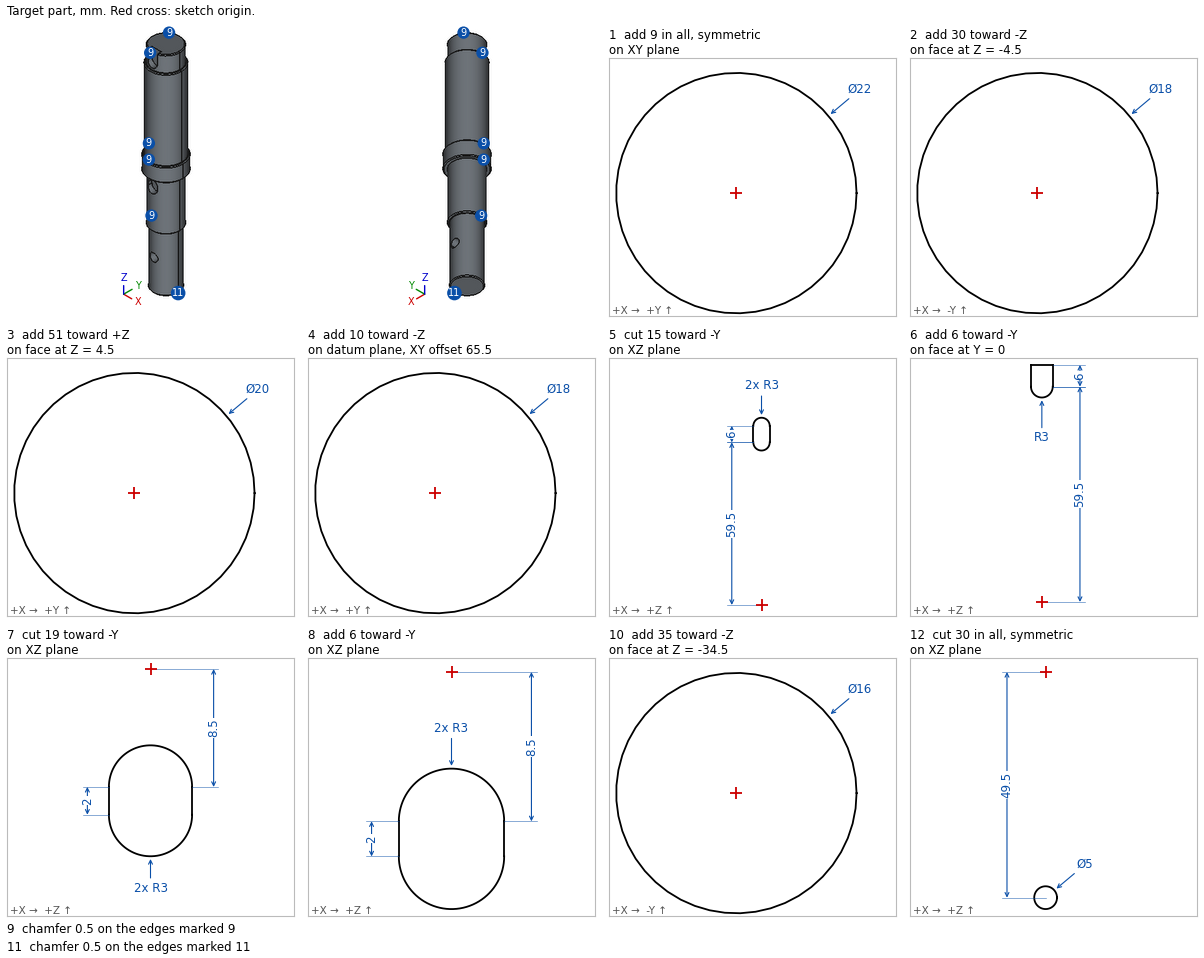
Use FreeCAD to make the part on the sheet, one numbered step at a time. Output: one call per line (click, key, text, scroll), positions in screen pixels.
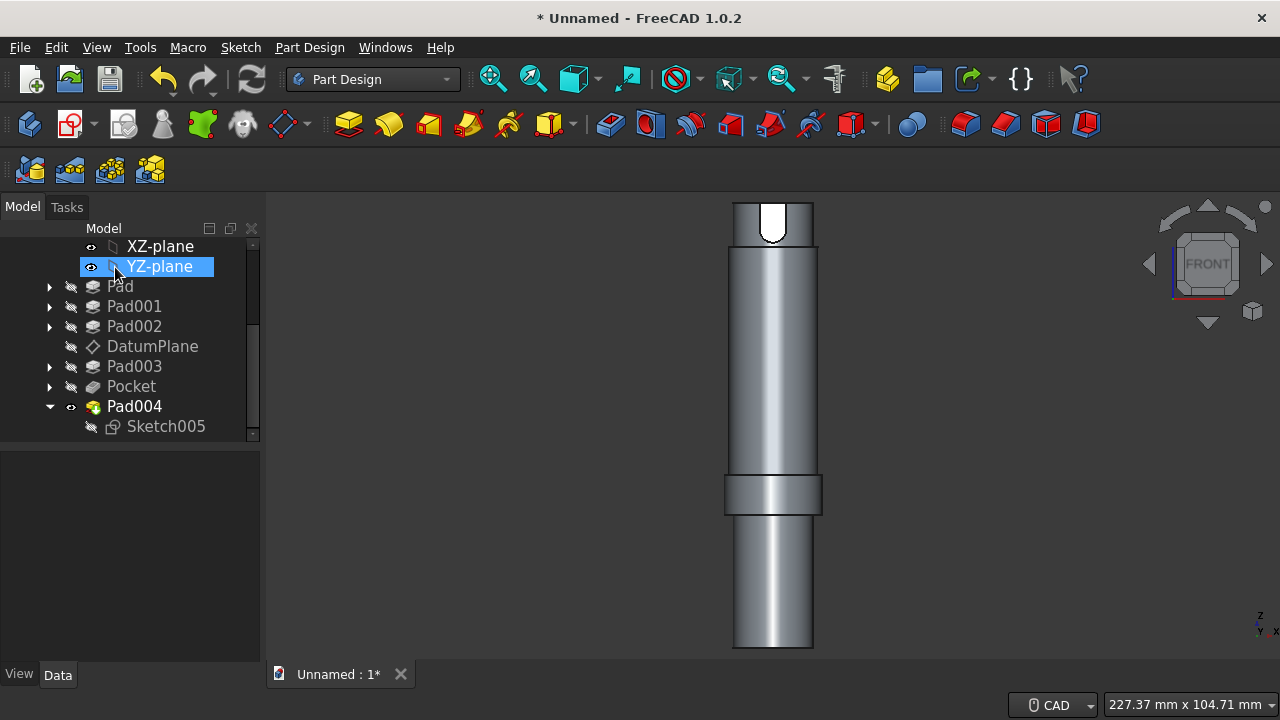
click(70, 124)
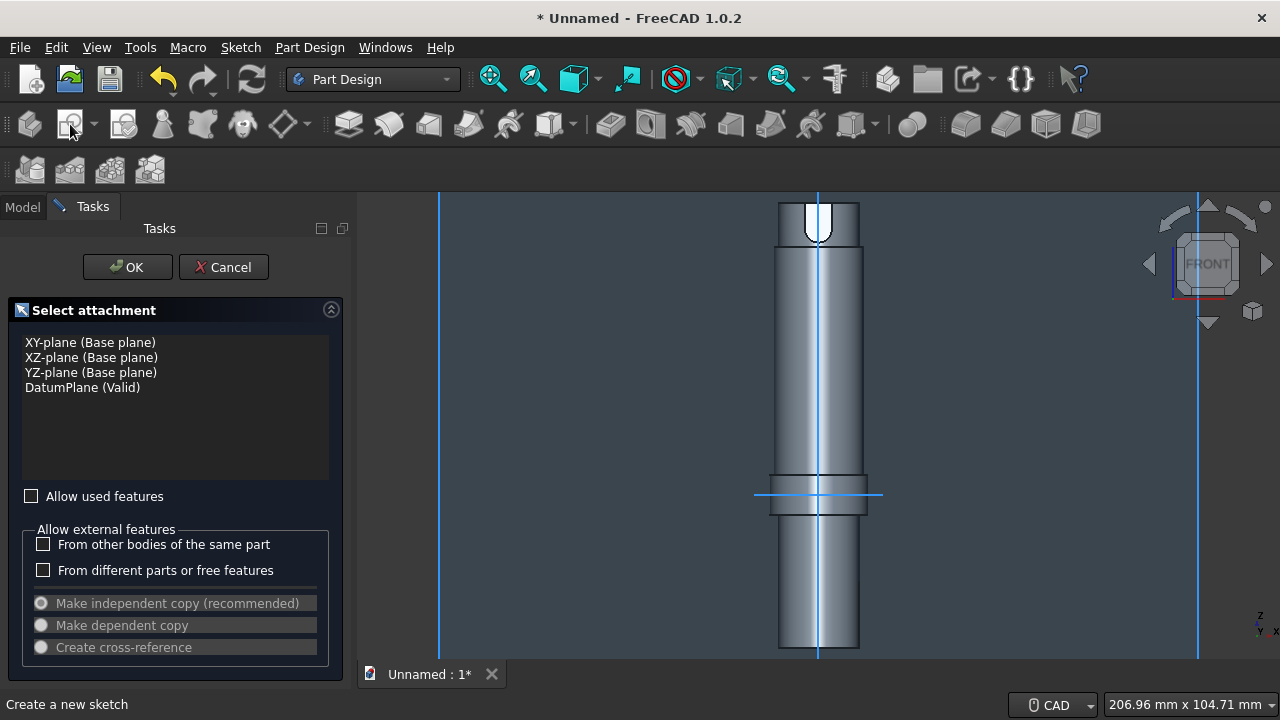
click(82, 358)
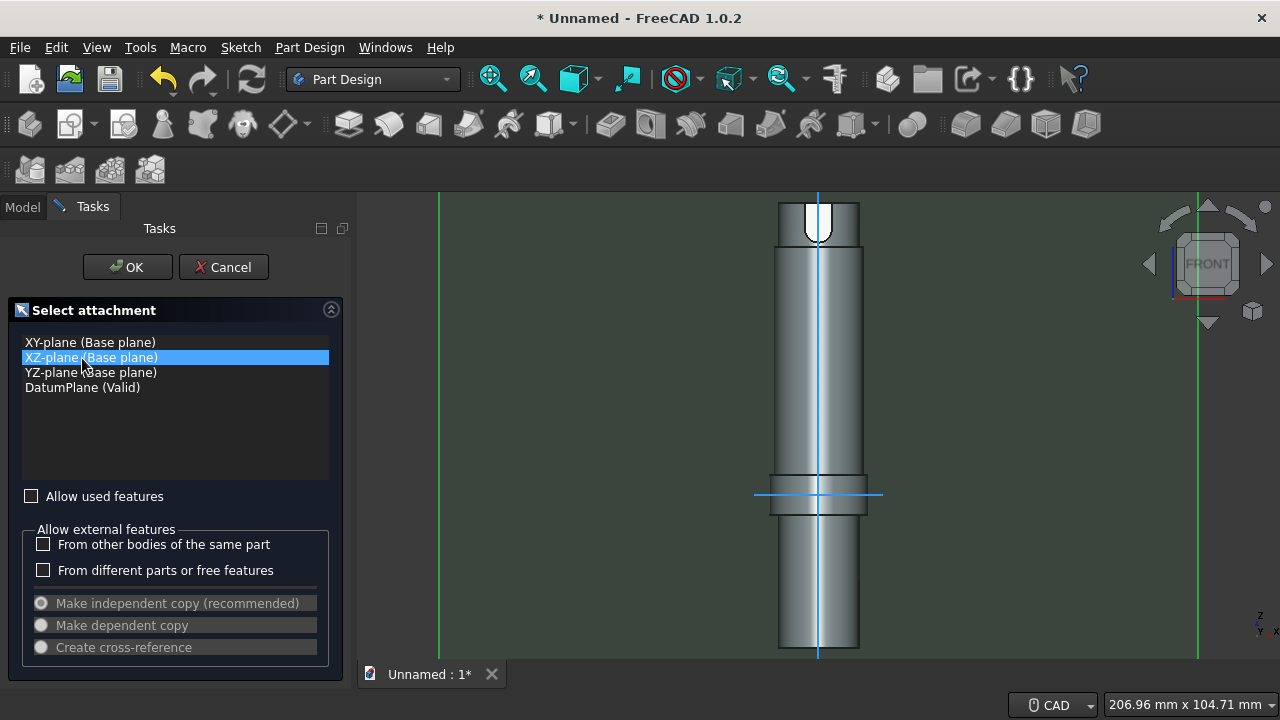
click(128, 267)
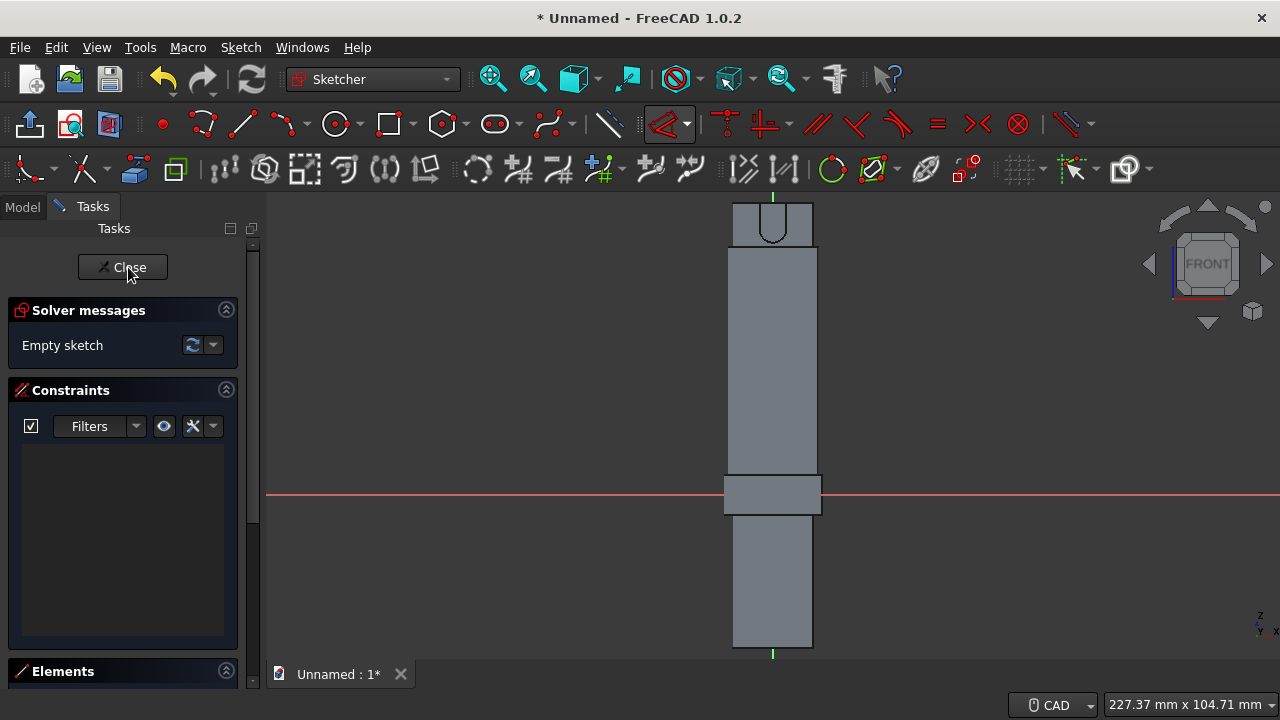
click(110, 124)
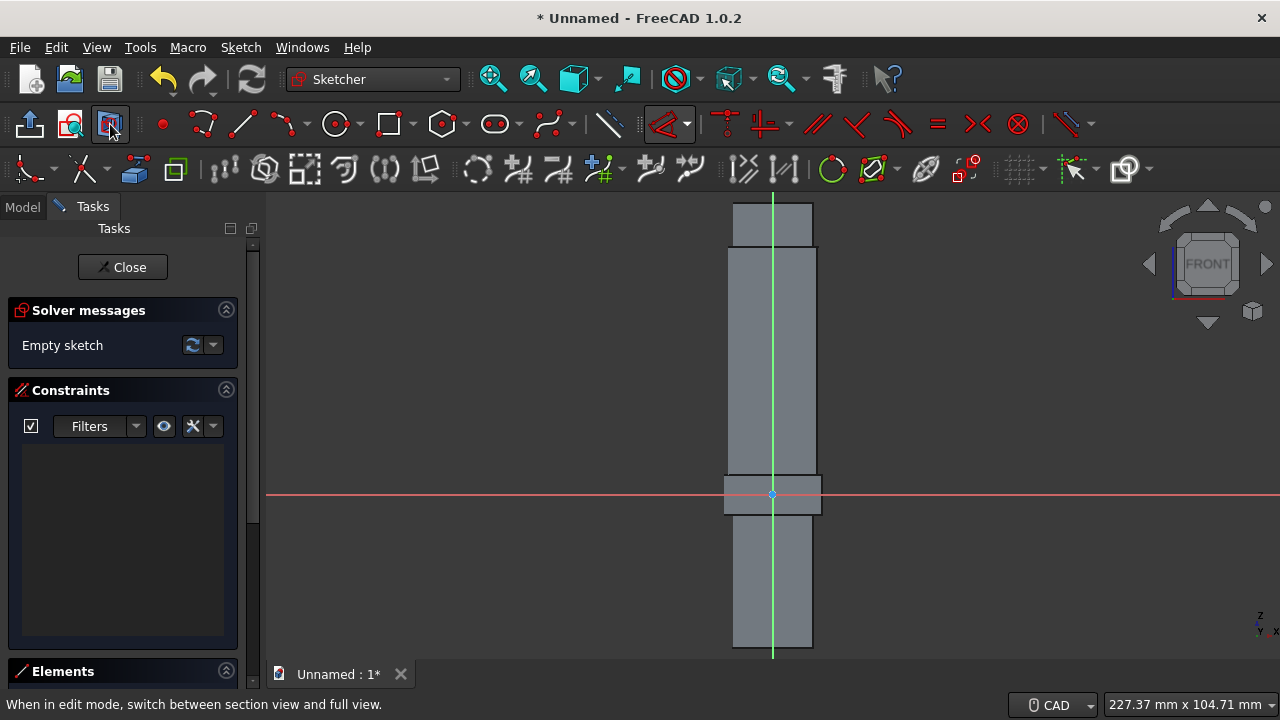
scroll(790, 550, up, 8)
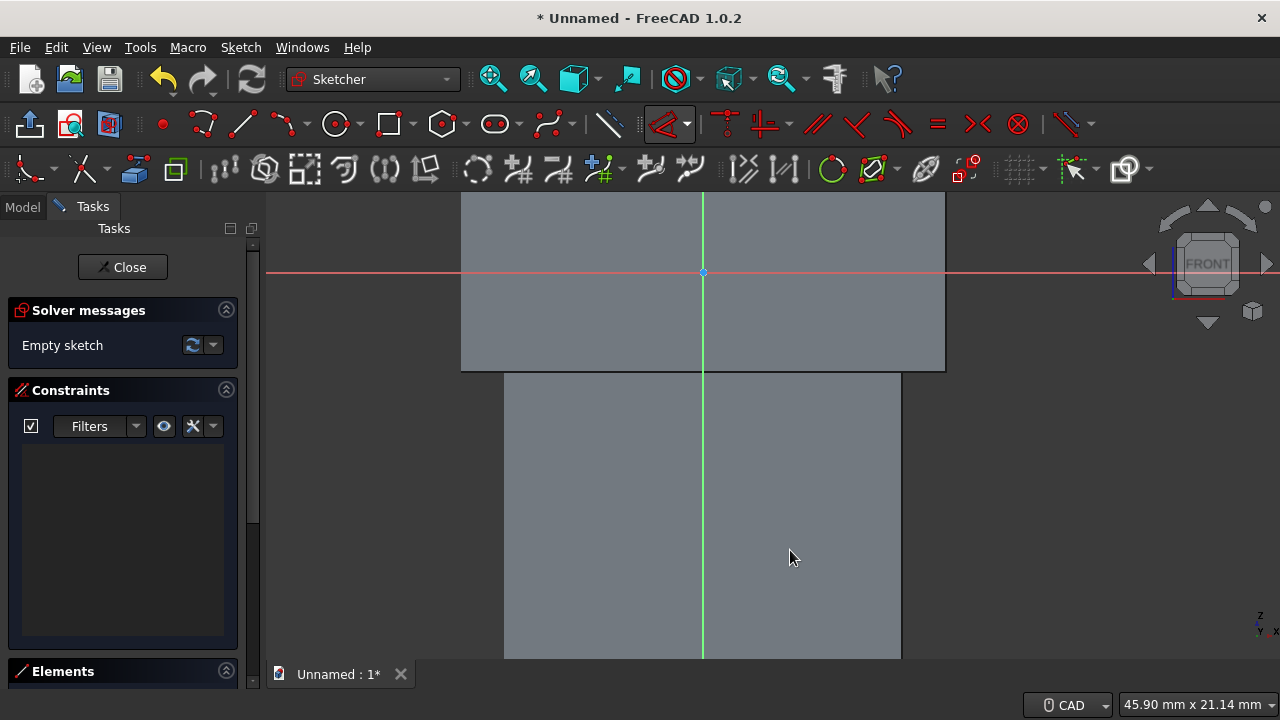
click(496, 124)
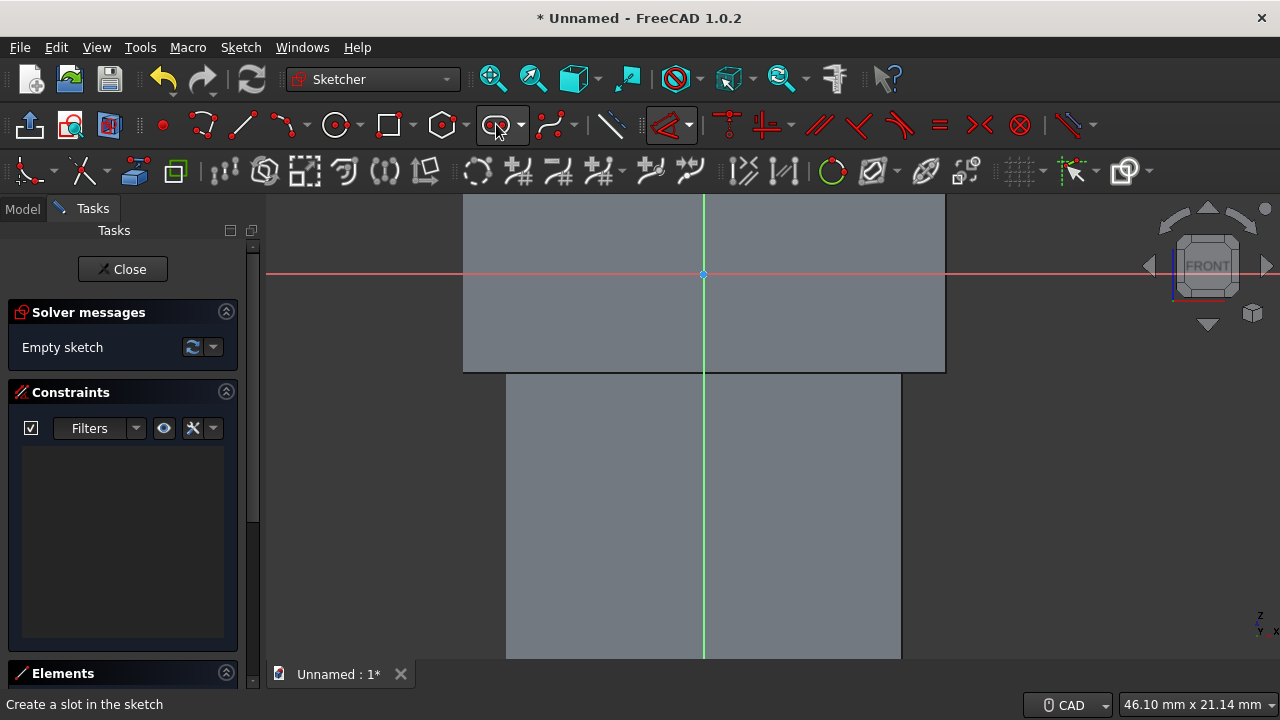
click(704, 505)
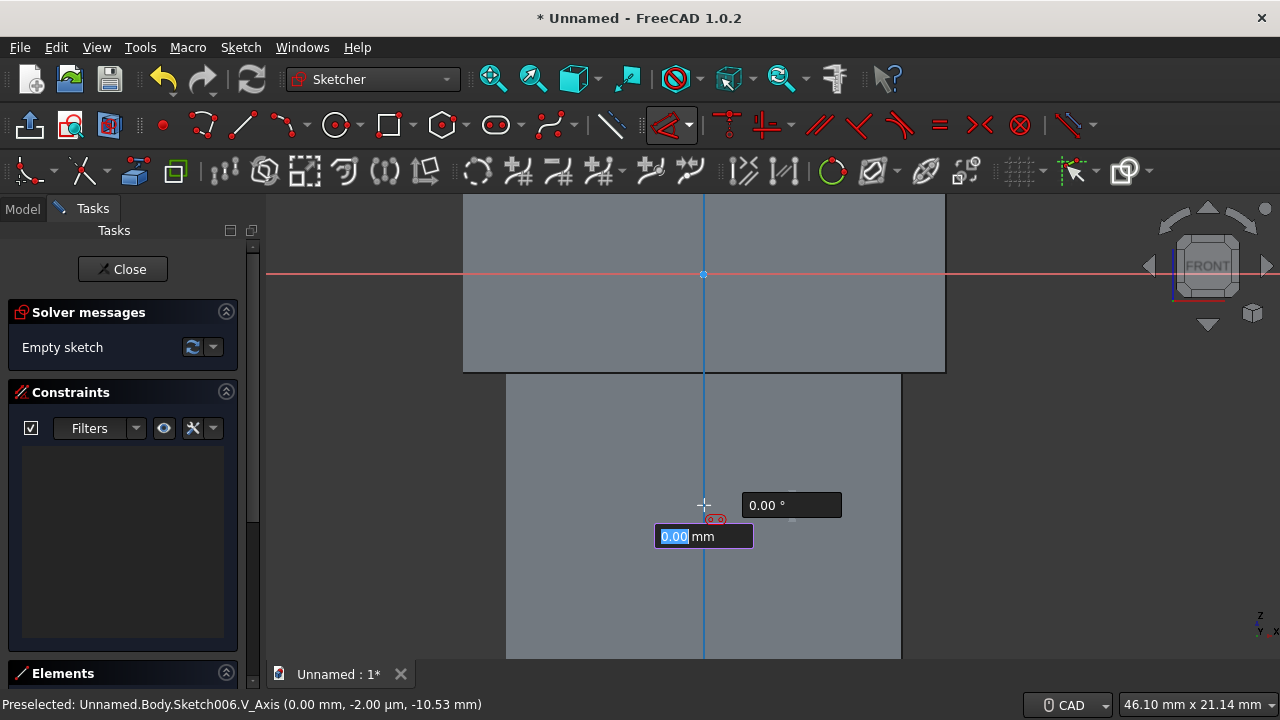
click(713, 461)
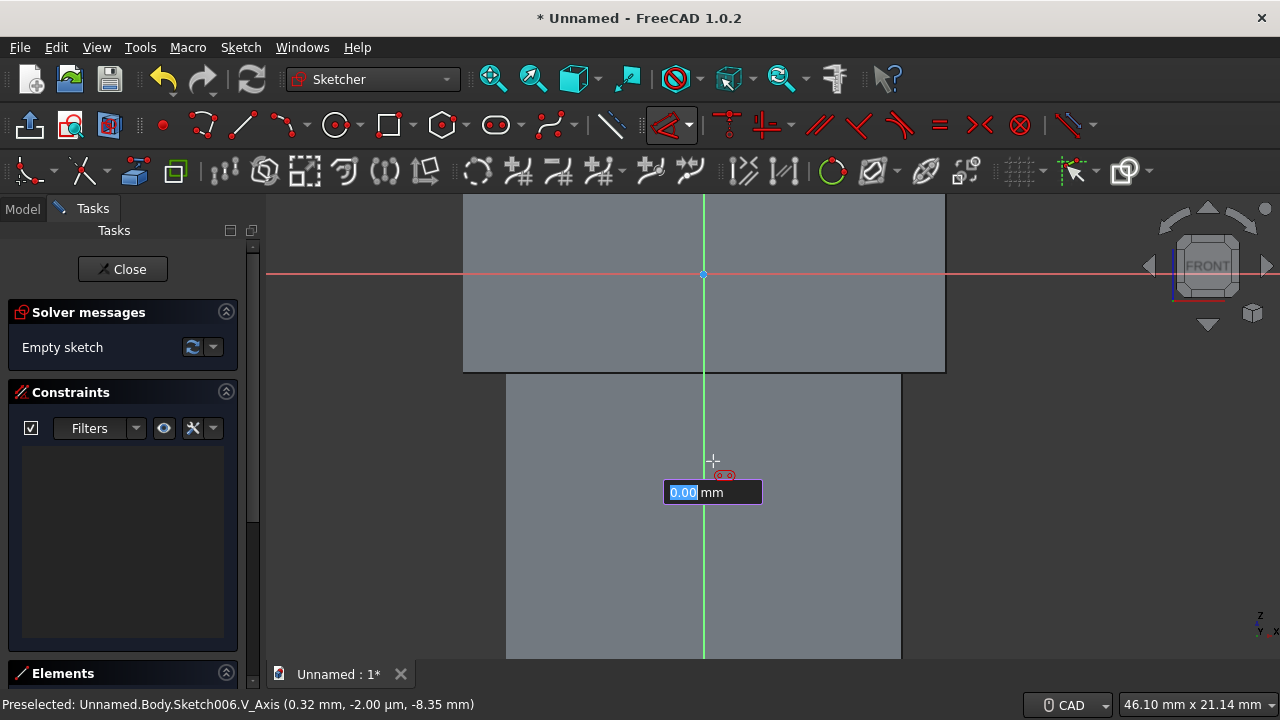
click(770, 483)
key(Escape)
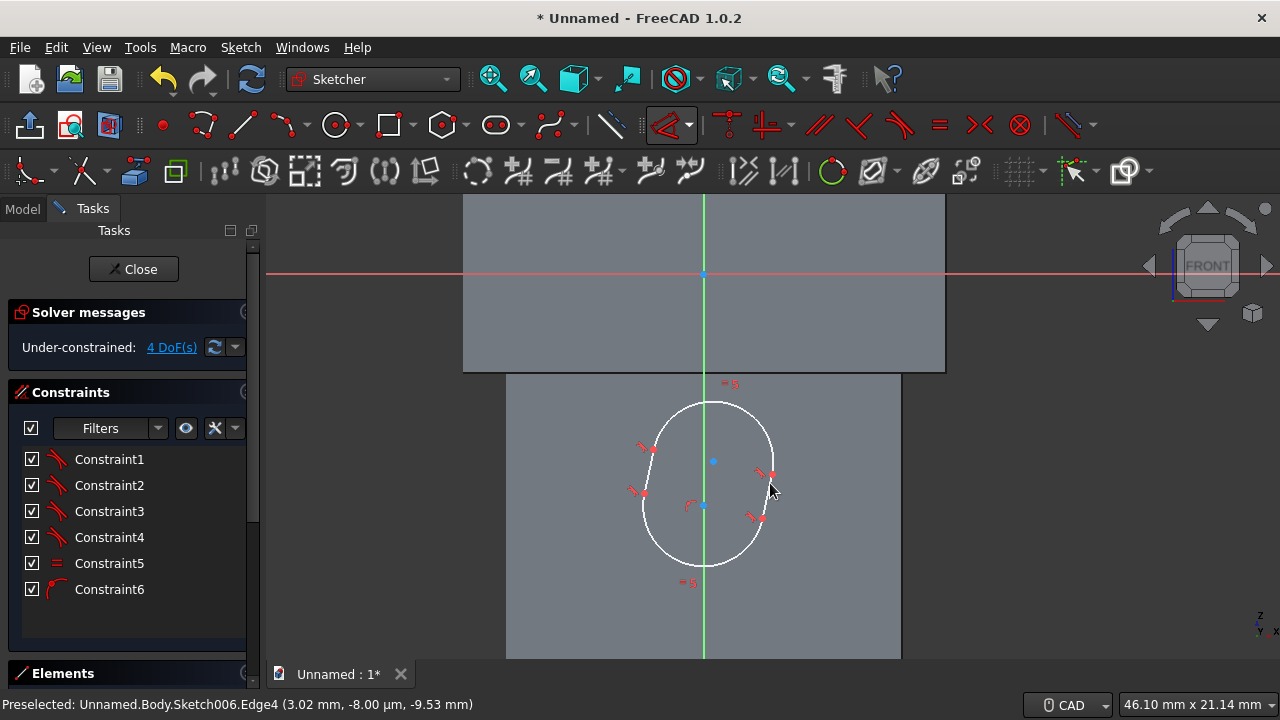
click(647, 480)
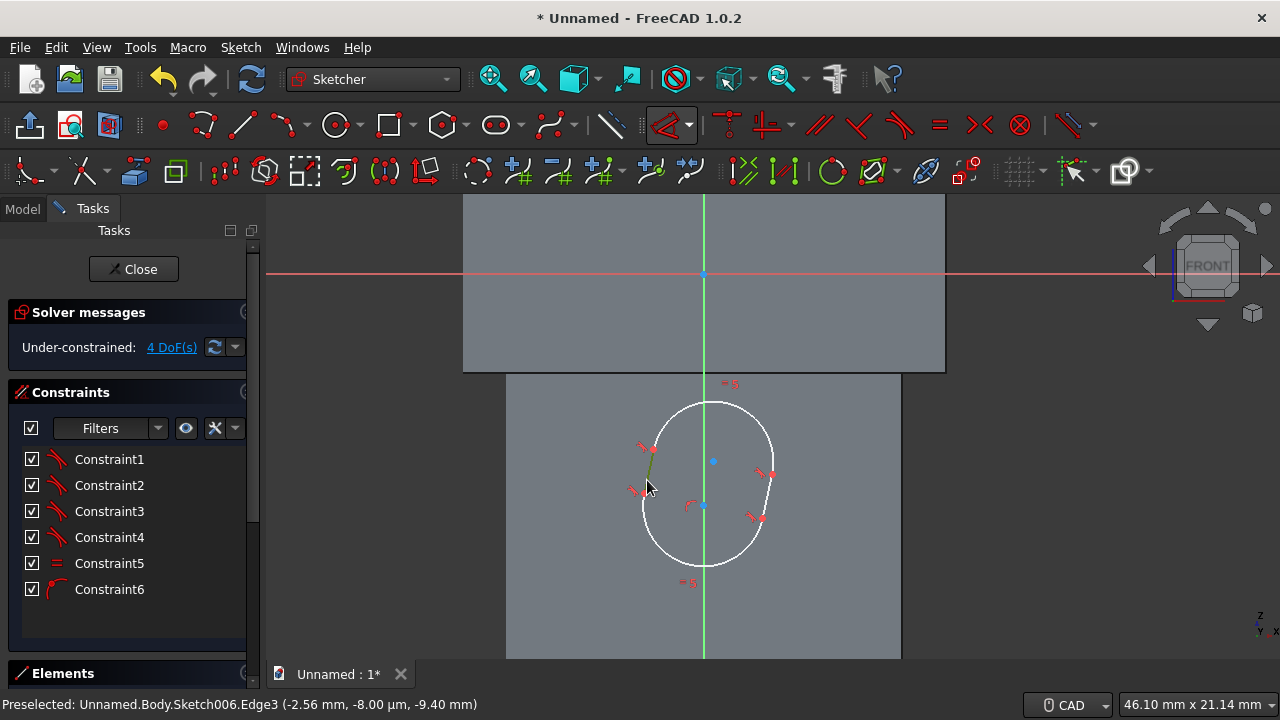
click(794, 126)